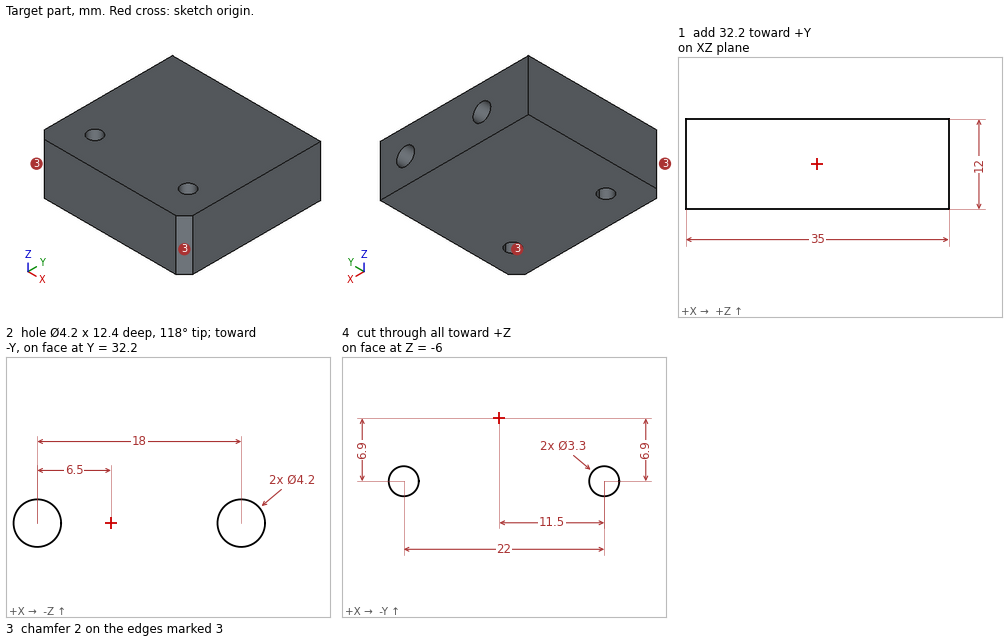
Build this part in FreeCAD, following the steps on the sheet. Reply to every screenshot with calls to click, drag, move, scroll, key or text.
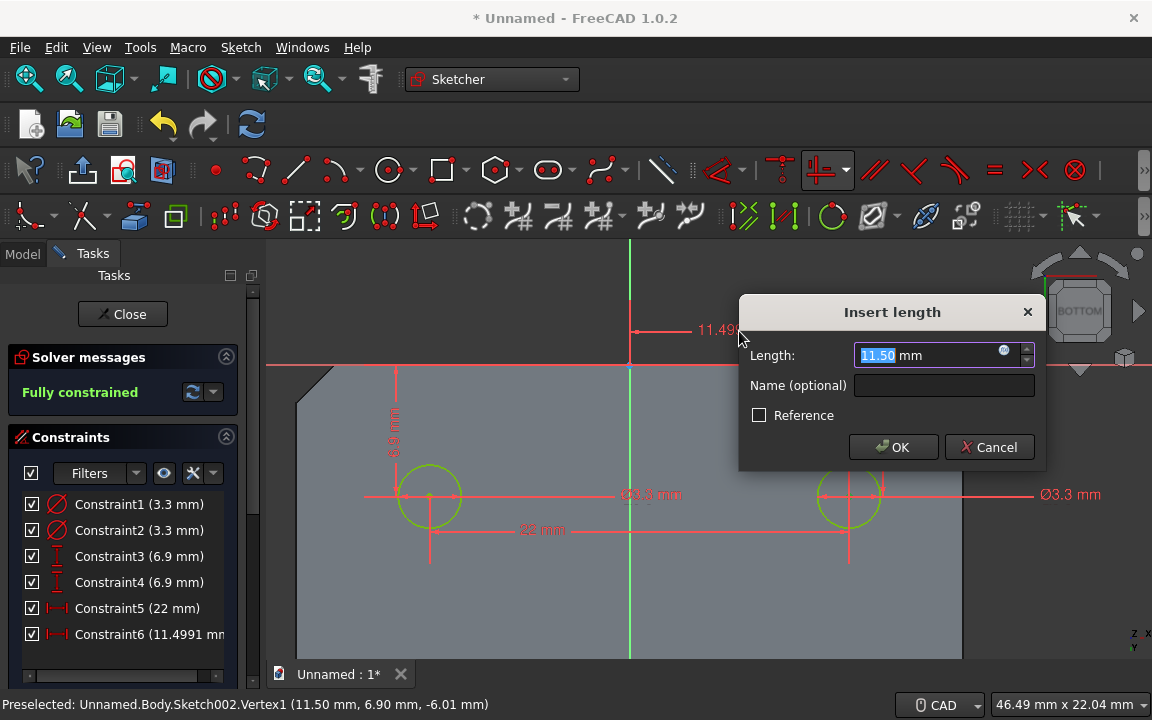
text(11.5)
key(Return)
key(Escape)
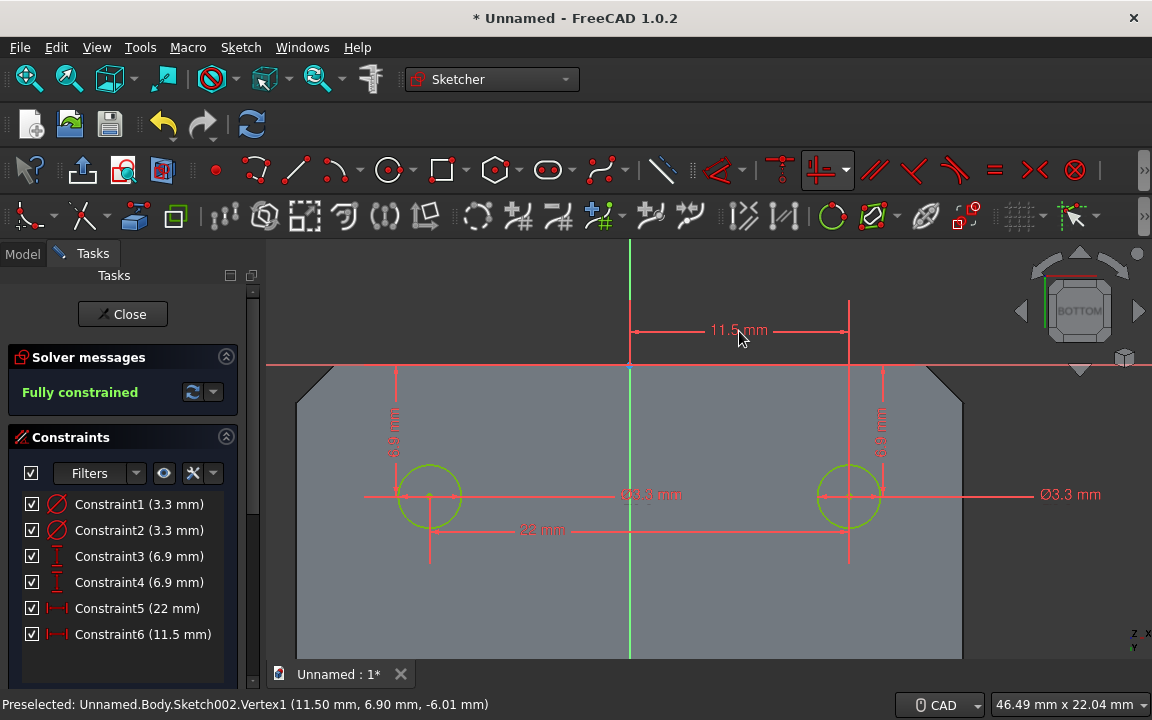
click(123, 314)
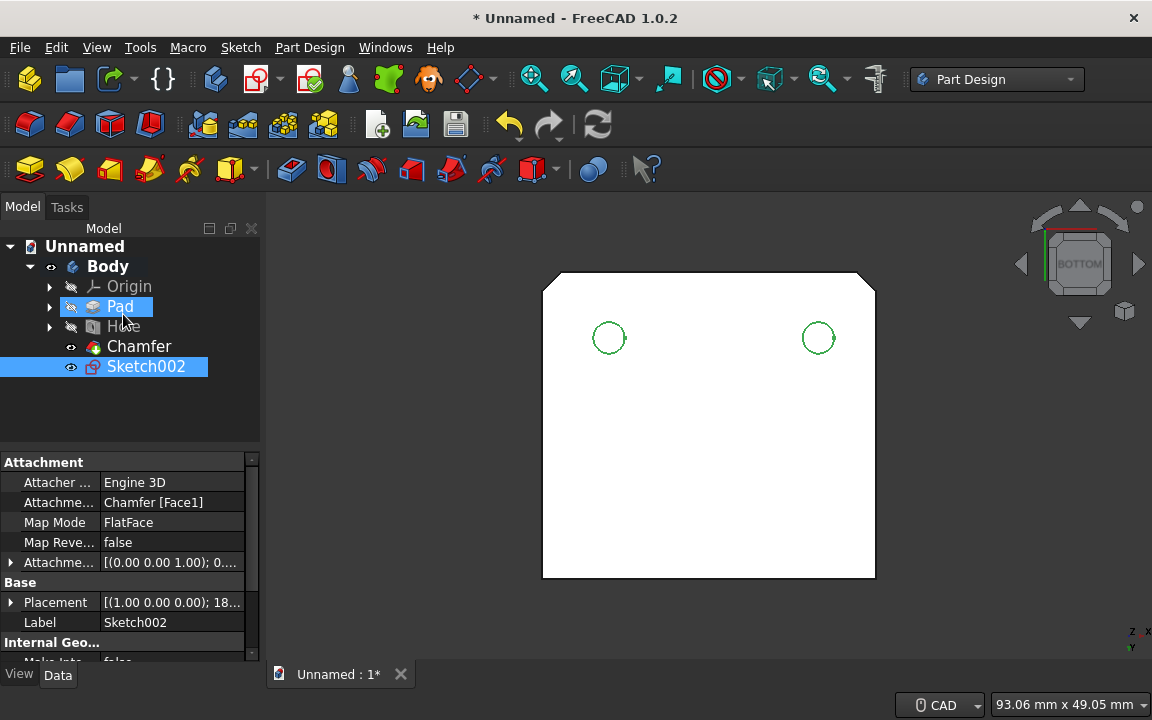
click(292, 170)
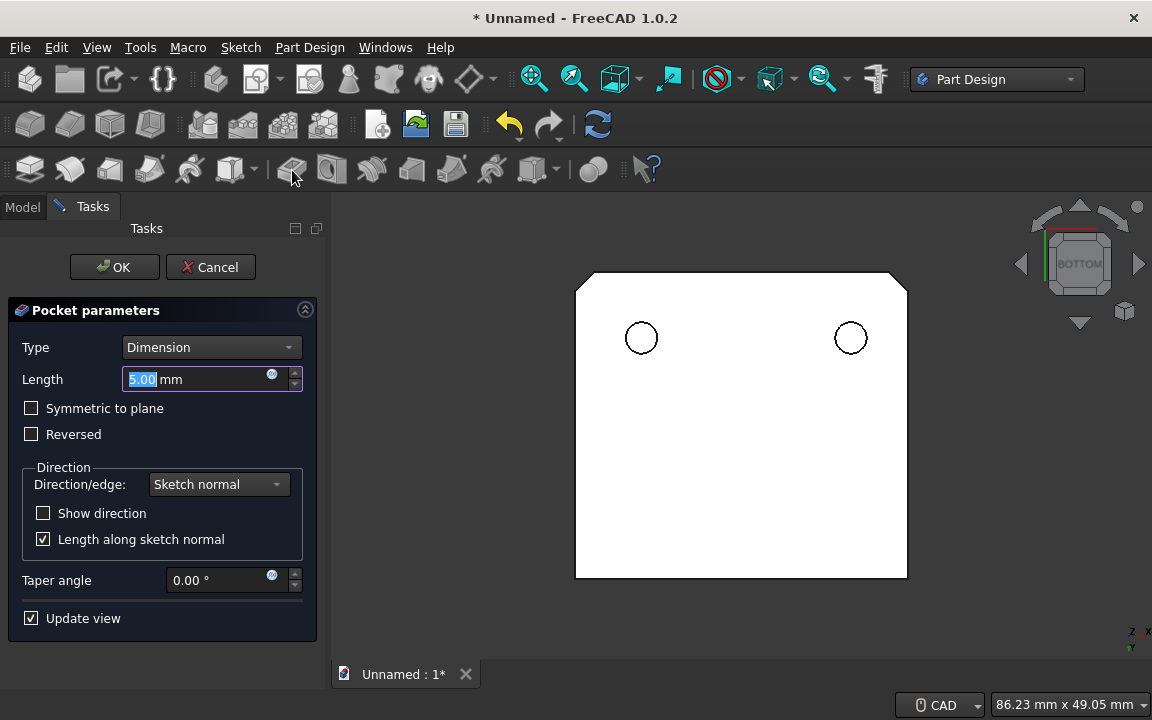
click(212, 348)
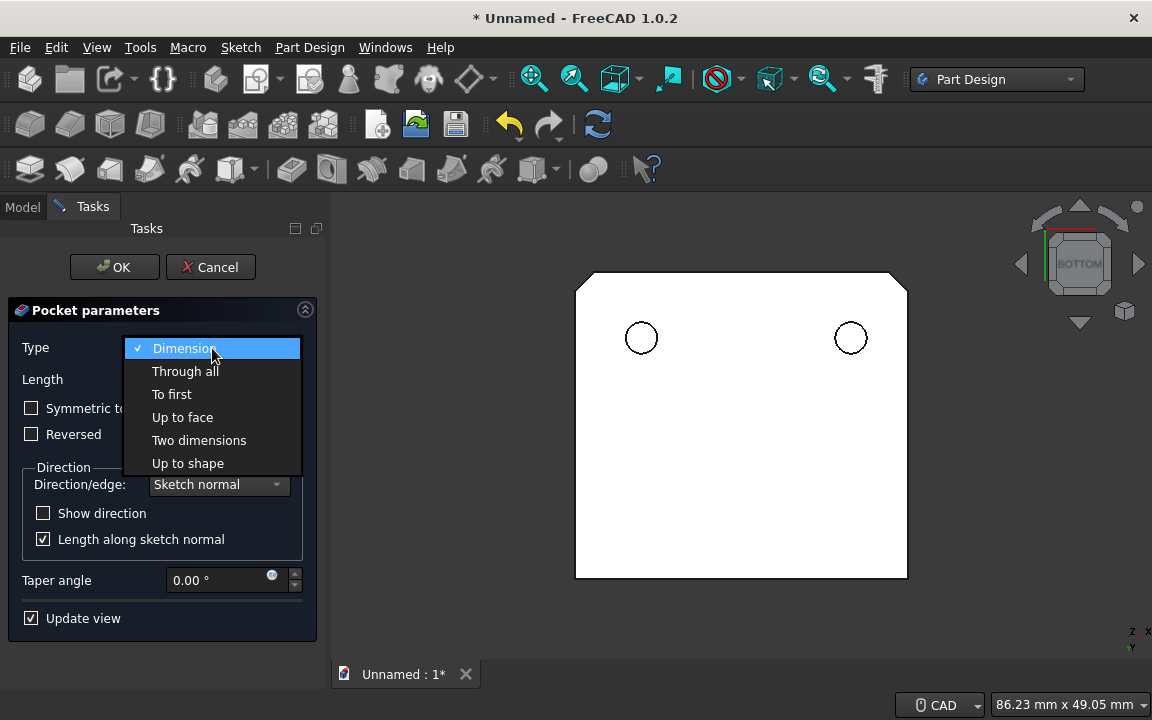
click(212, 372)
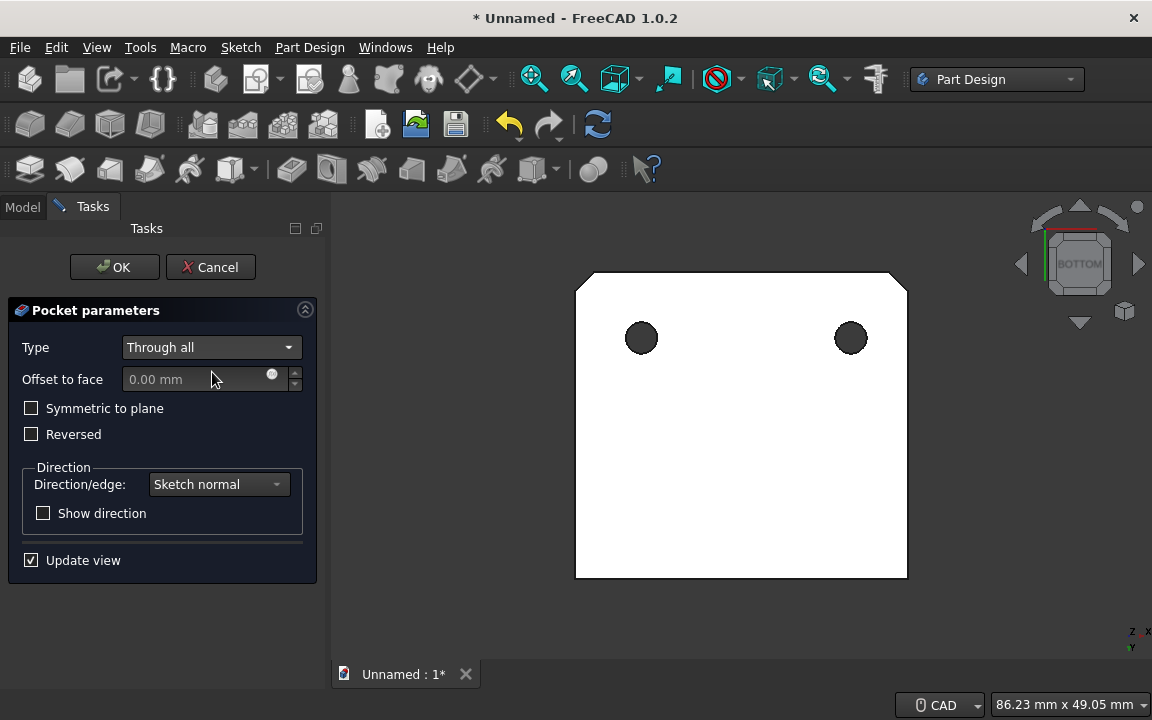
click(115, 267)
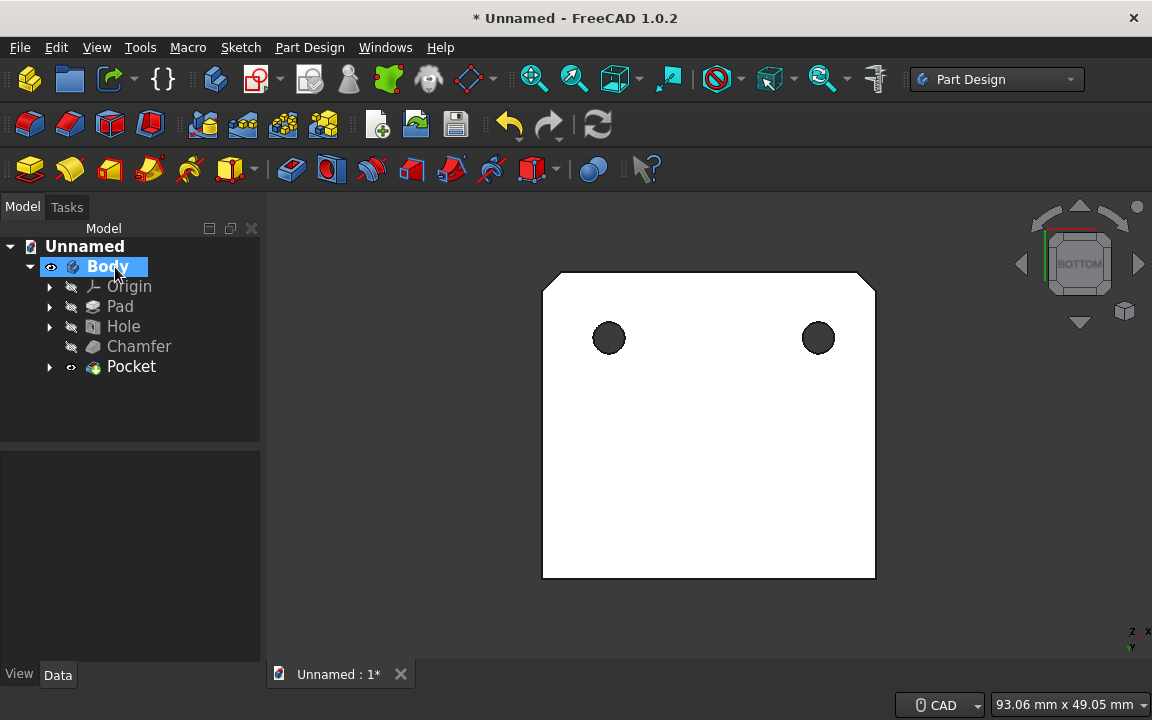
key(0)